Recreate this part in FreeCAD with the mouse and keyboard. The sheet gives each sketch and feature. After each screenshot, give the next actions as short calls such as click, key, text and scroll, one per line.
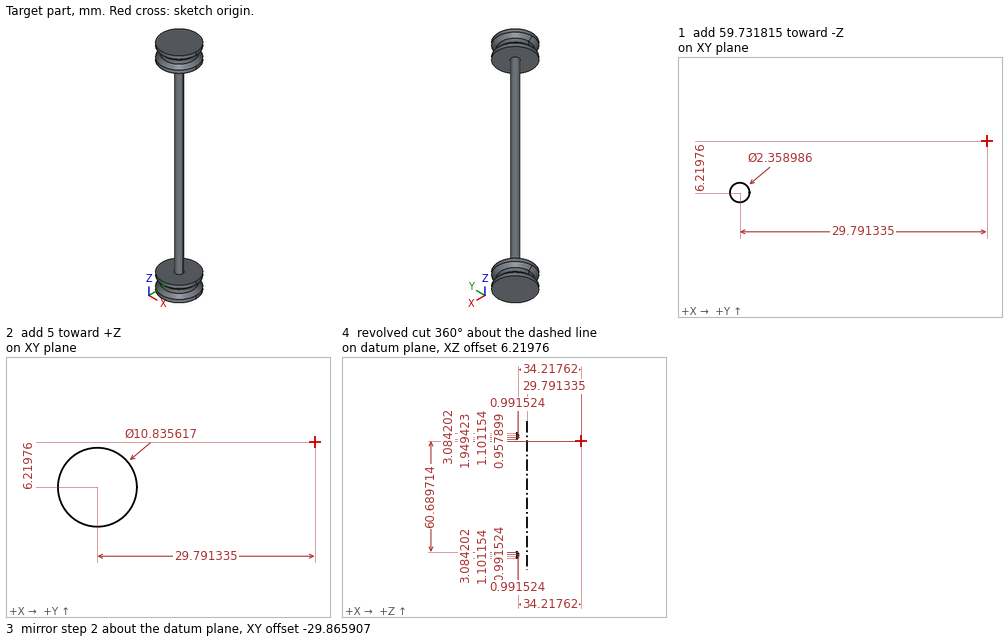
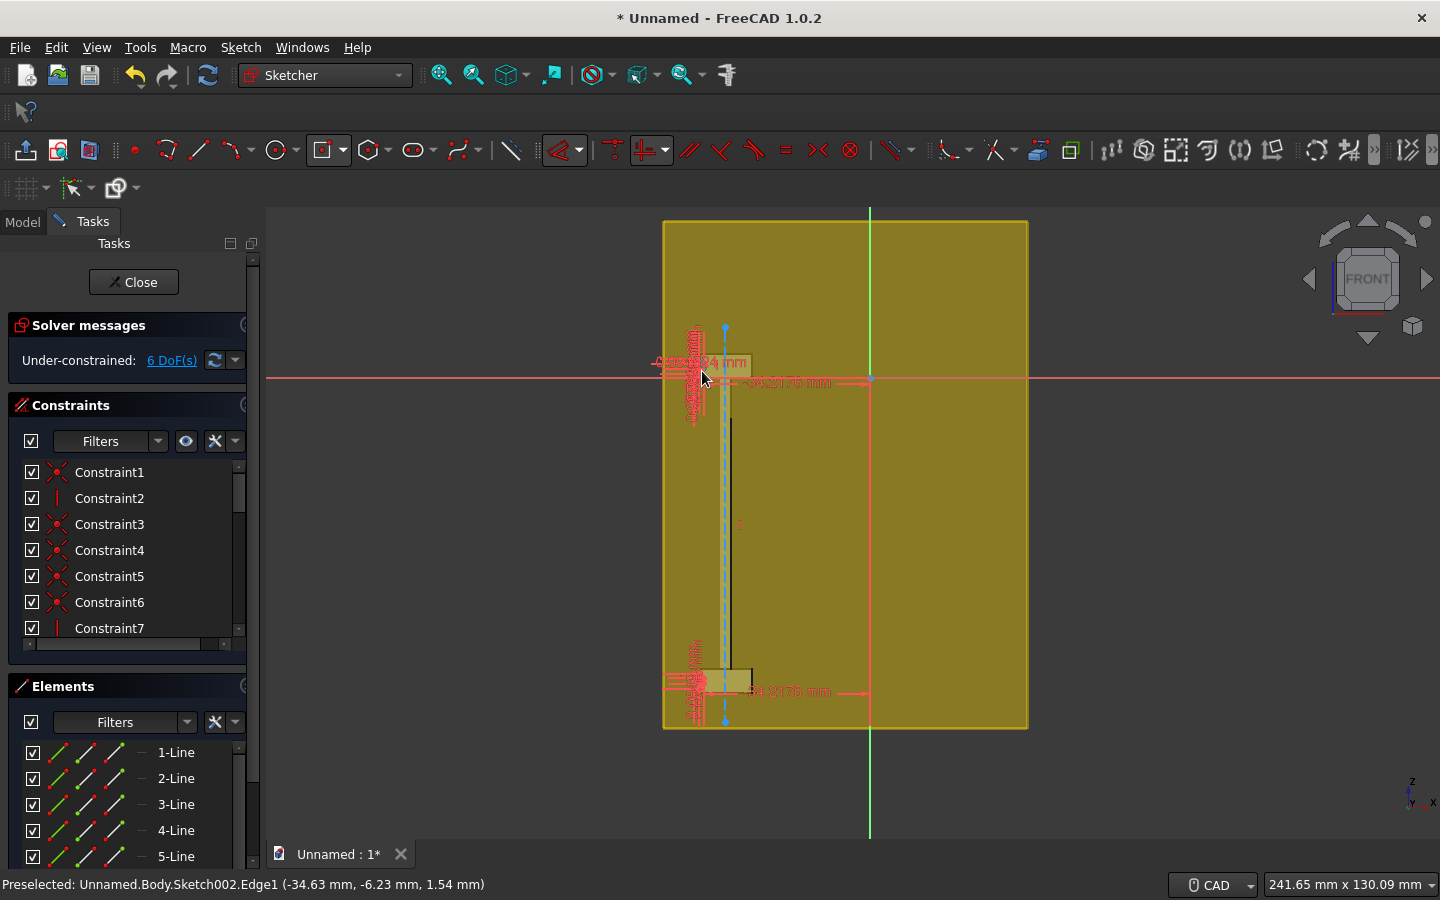
scroll(701, 675, up, 12)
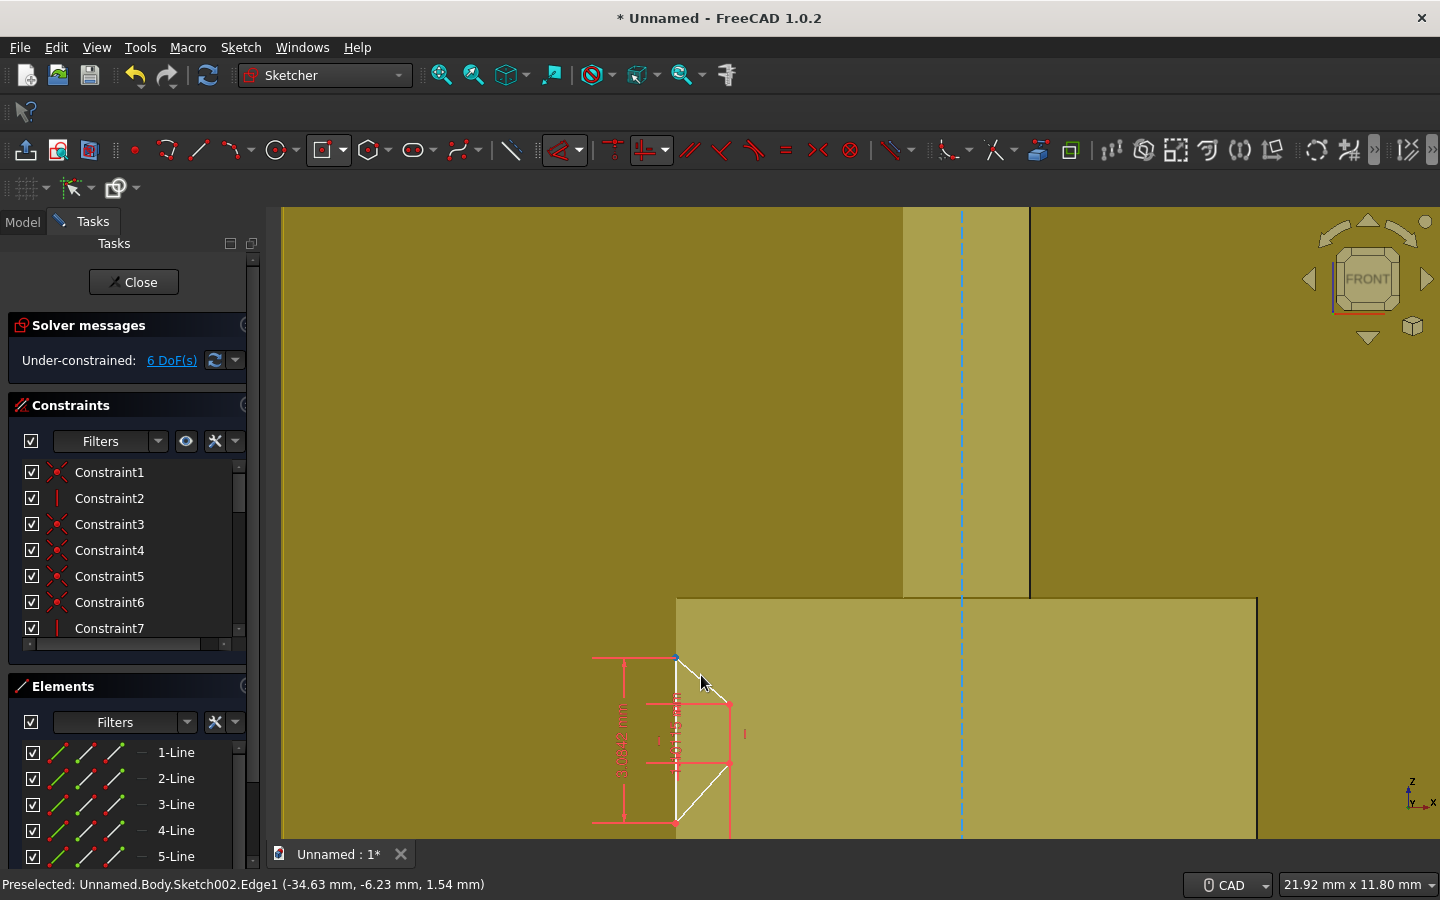
click(692, 672)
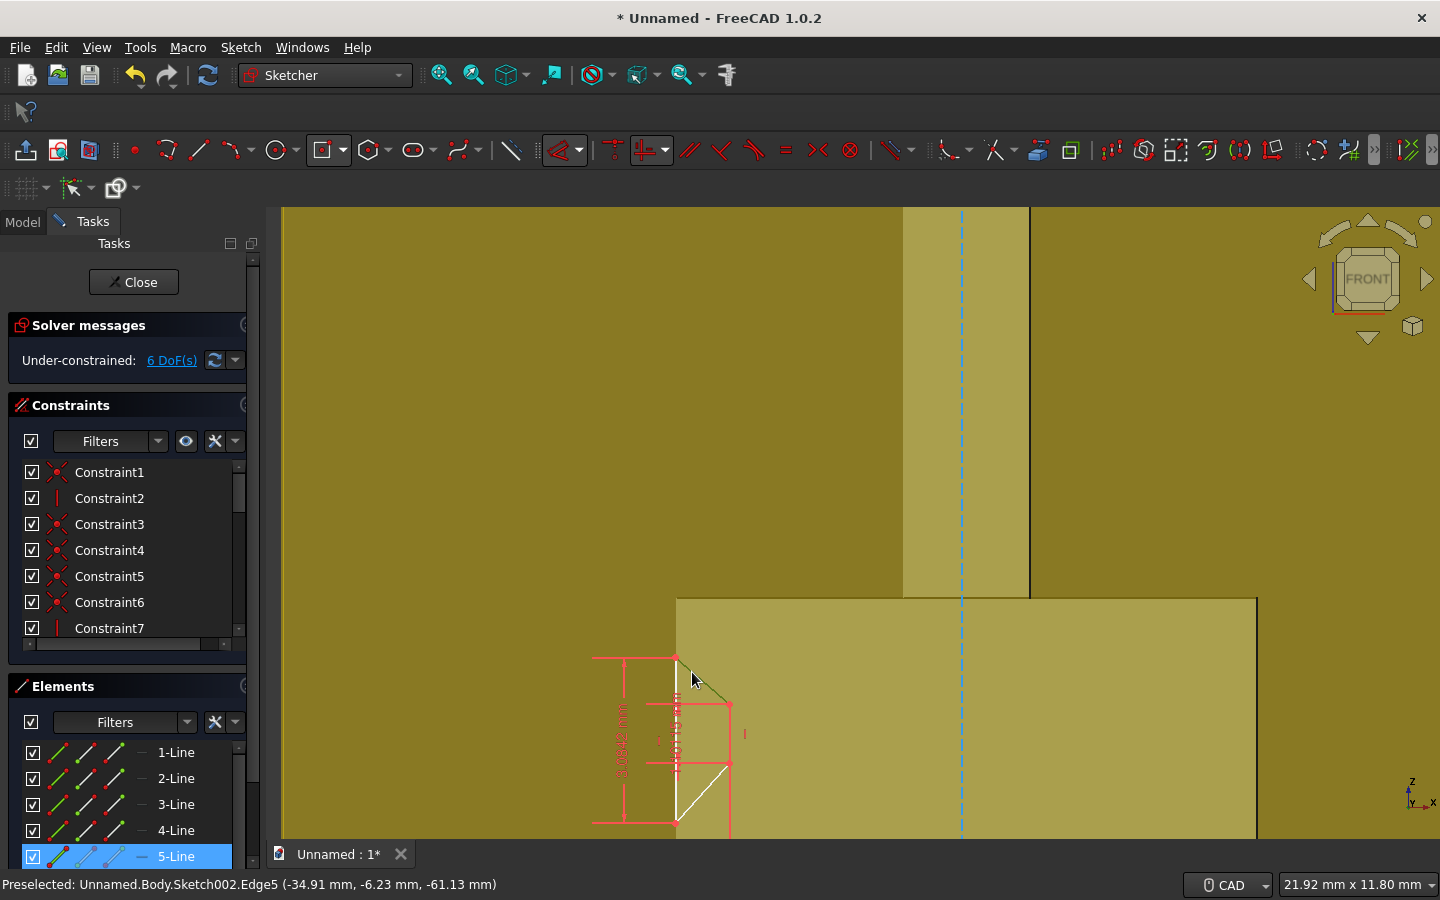
click(582, 150)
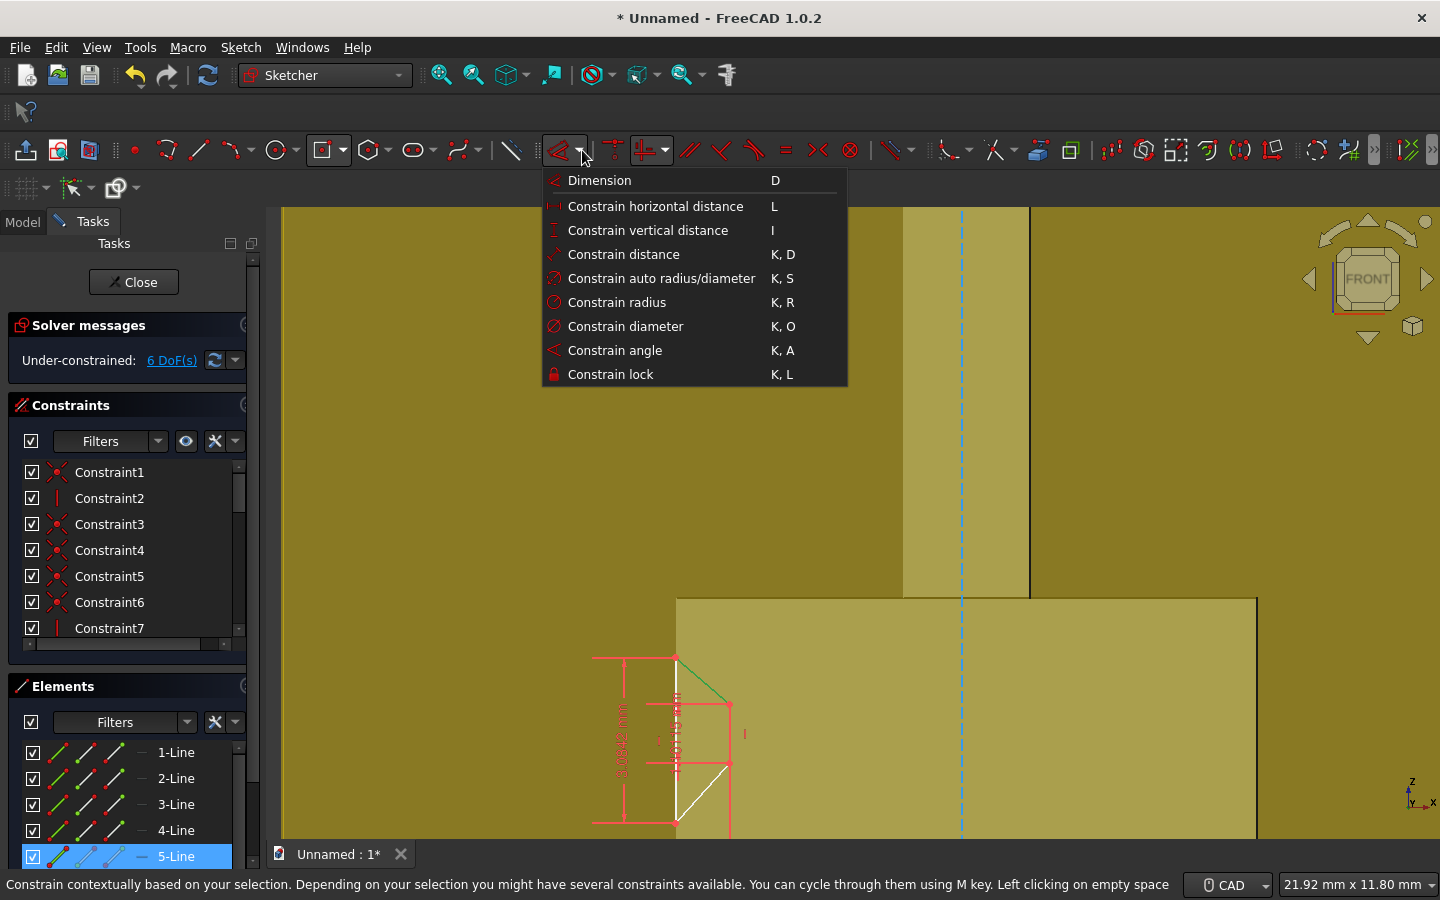
click(695, 206)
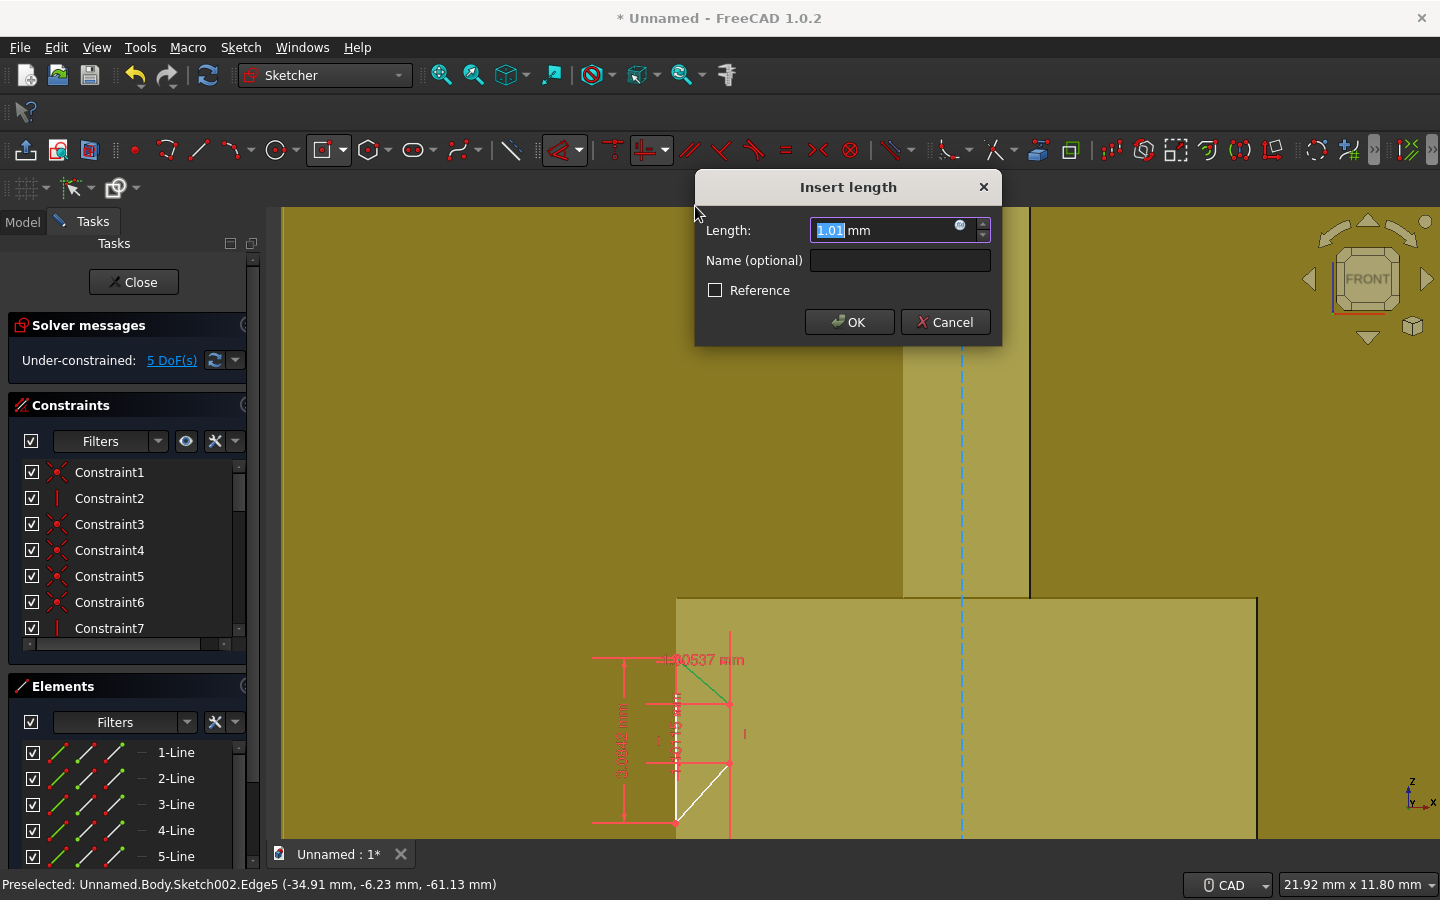
text(0.991524)
key(Return)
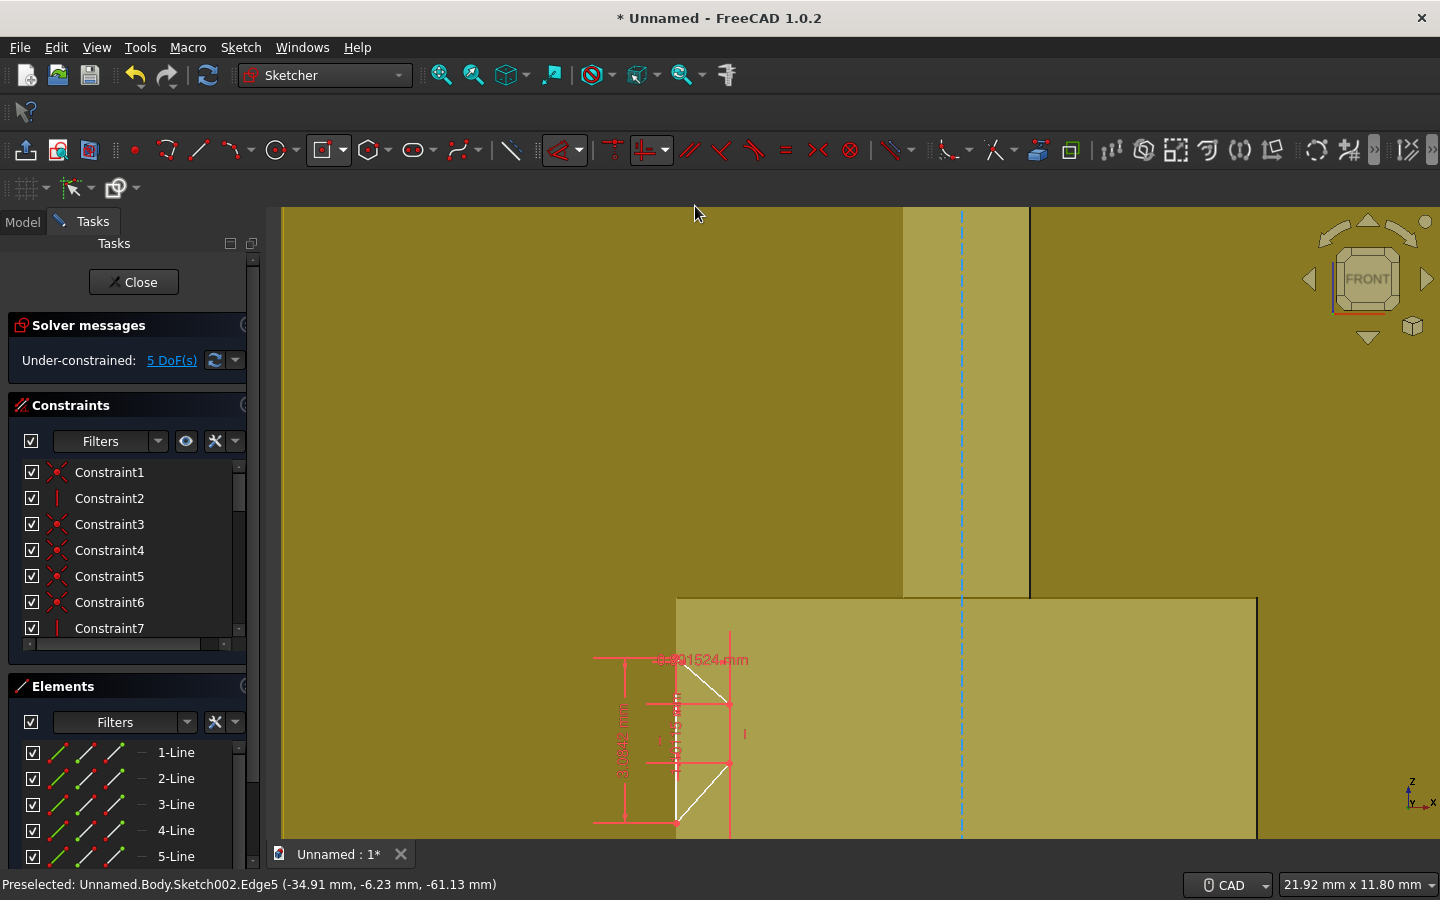
click(692, 672)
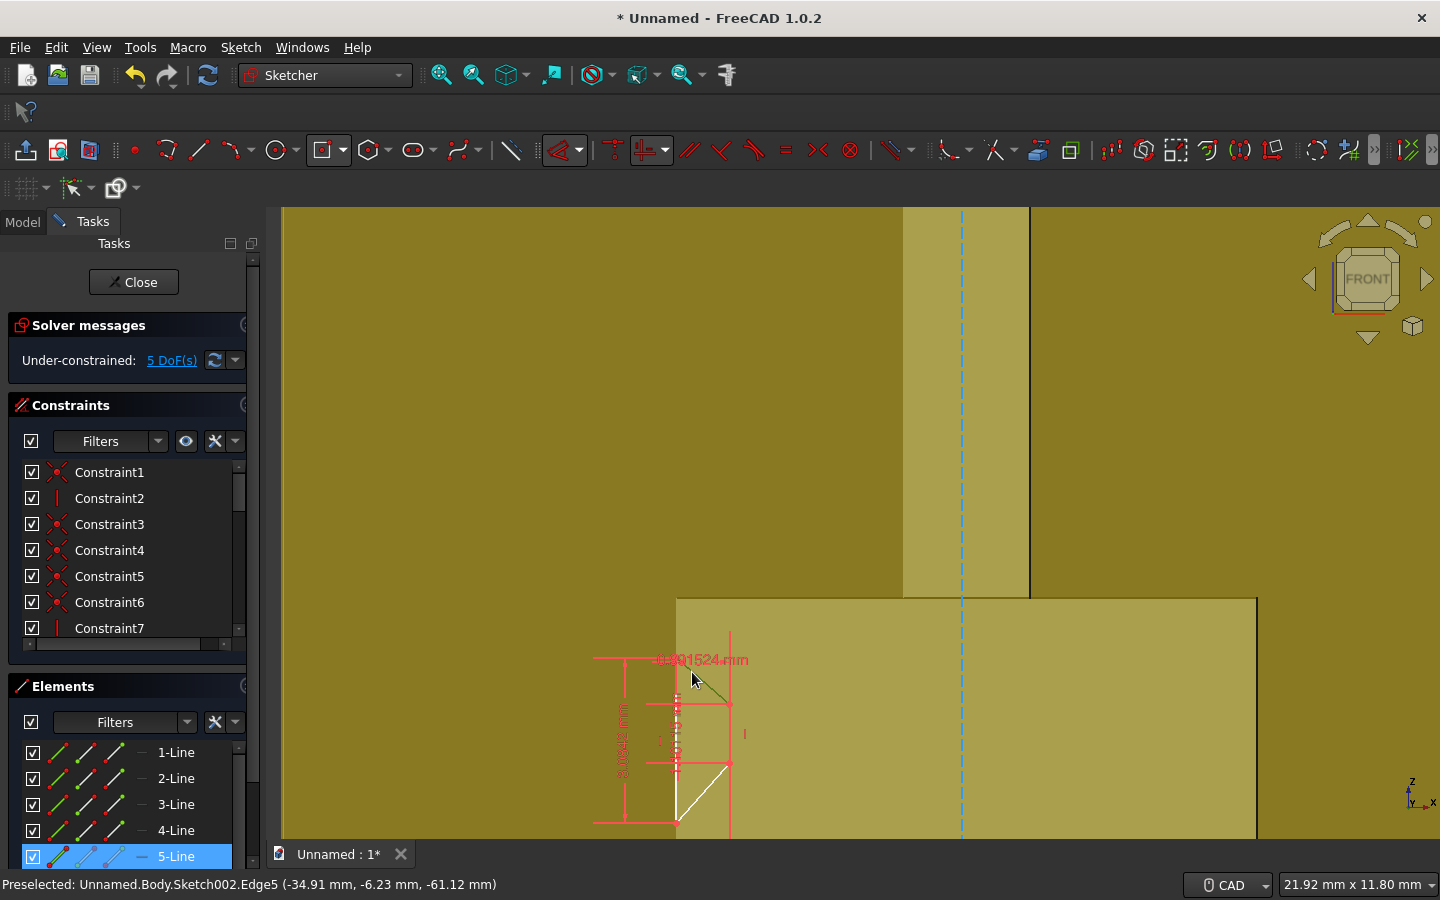
key(i)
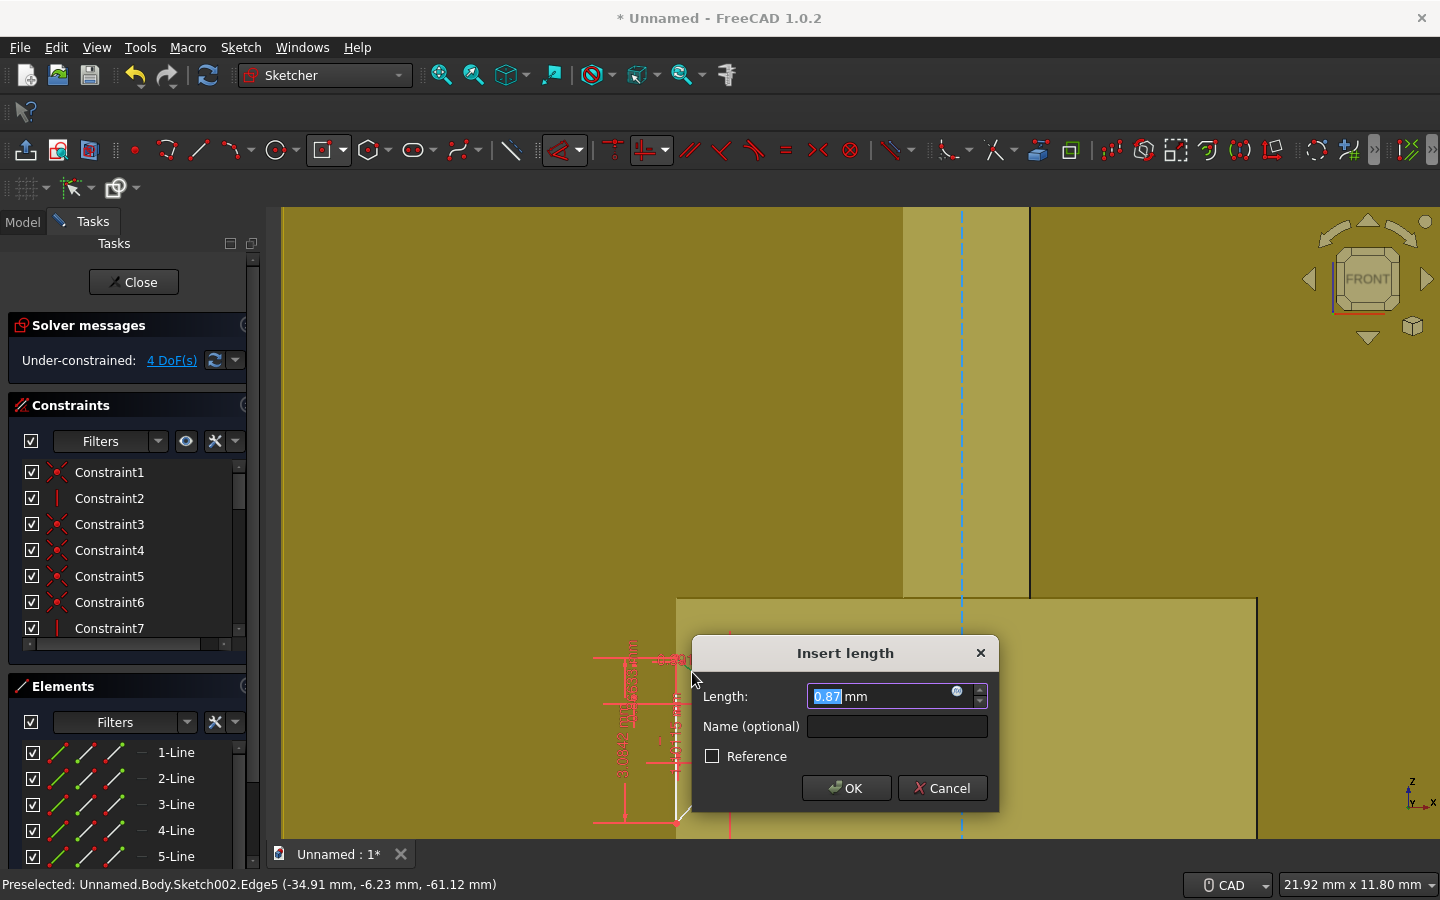
text(0.991524)
key(Return)